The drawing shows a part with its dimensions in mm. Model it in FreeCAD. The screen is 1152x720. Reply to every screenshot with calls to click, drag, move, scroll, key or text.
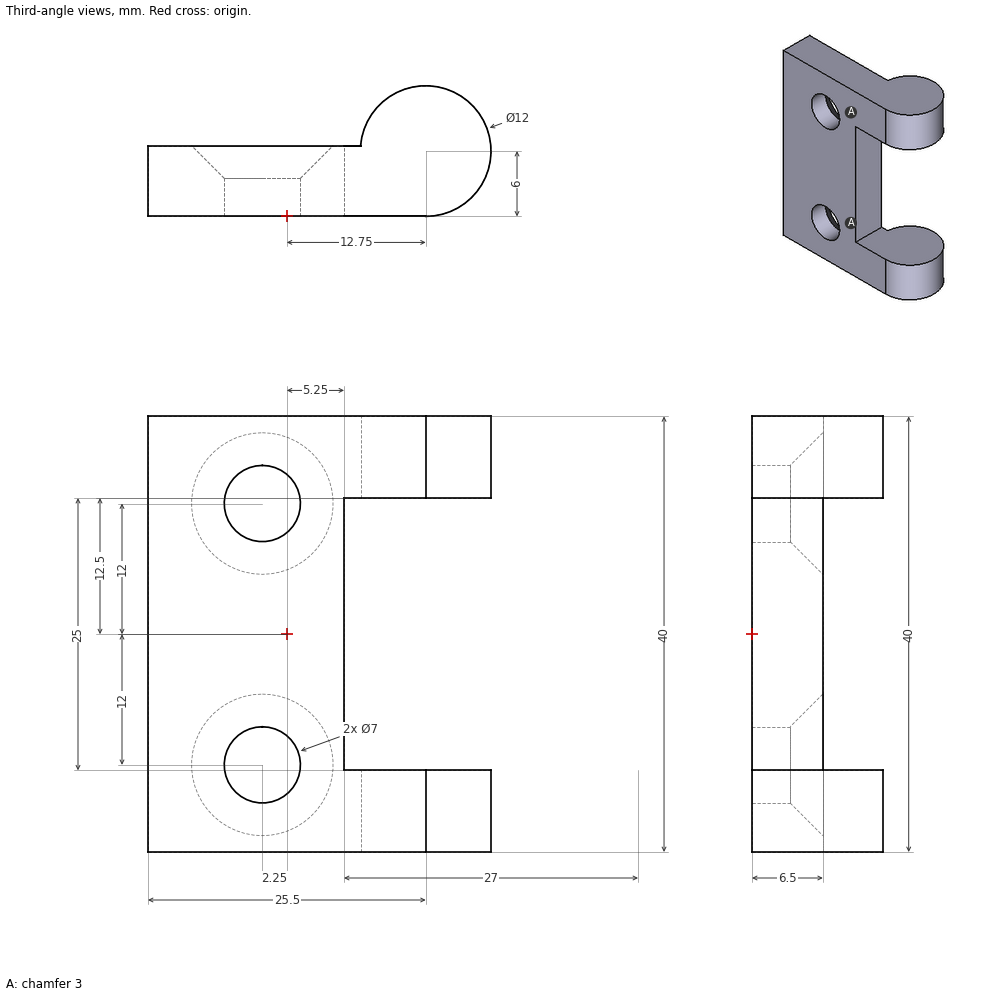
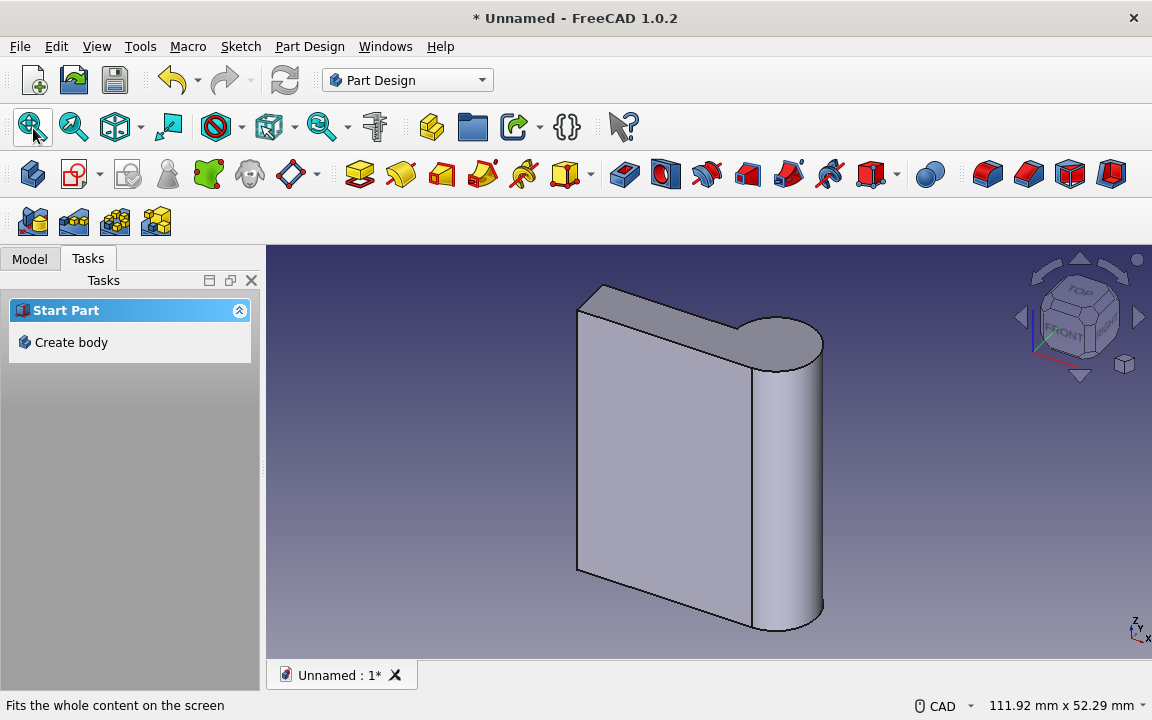
click(665, 431)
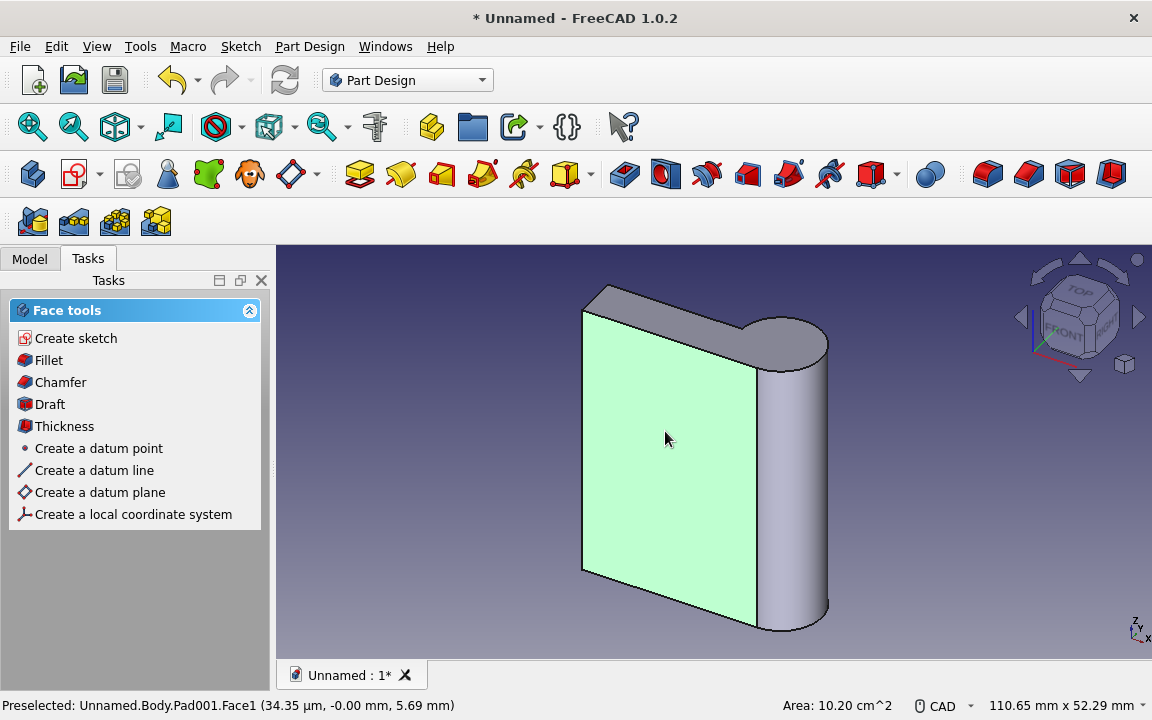
click(74, 174)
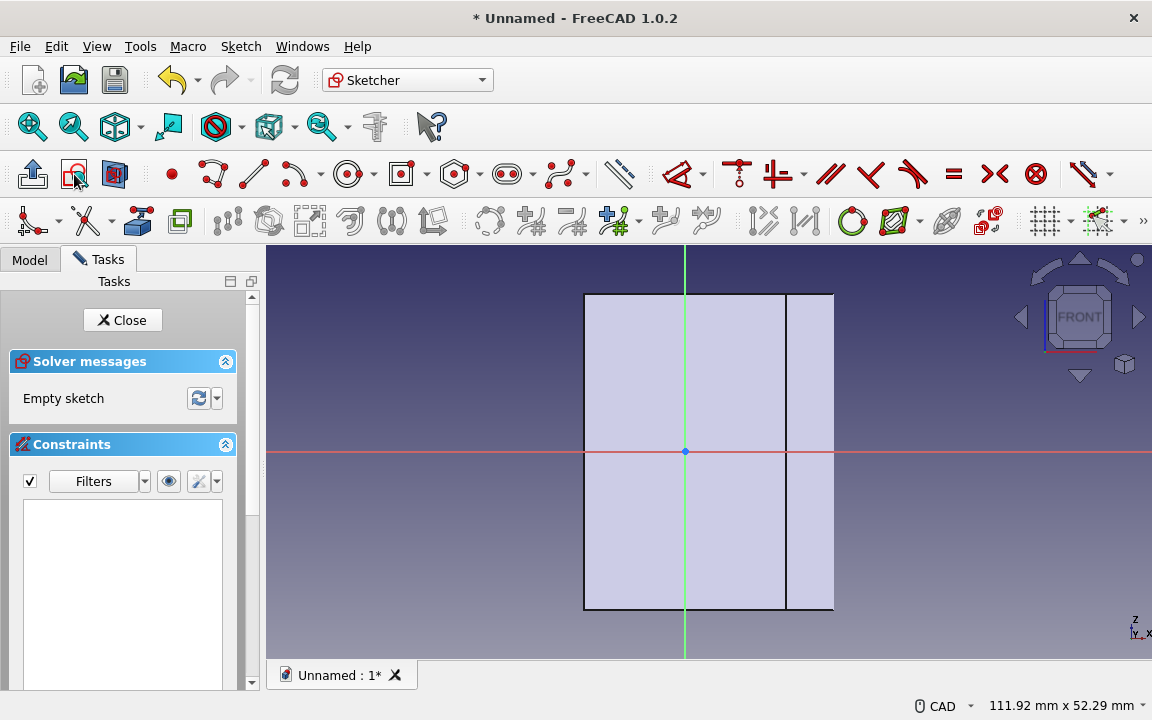
key(g)
key(r)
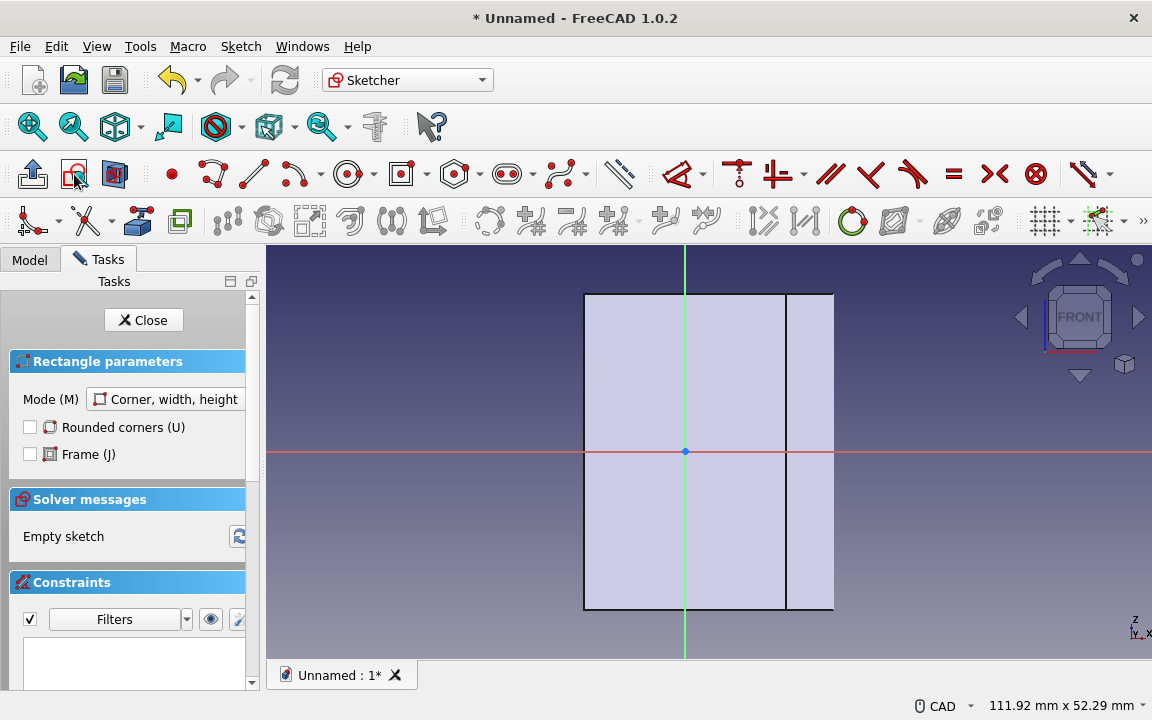
click(727, 353)
click(941, 551)
key(Escape)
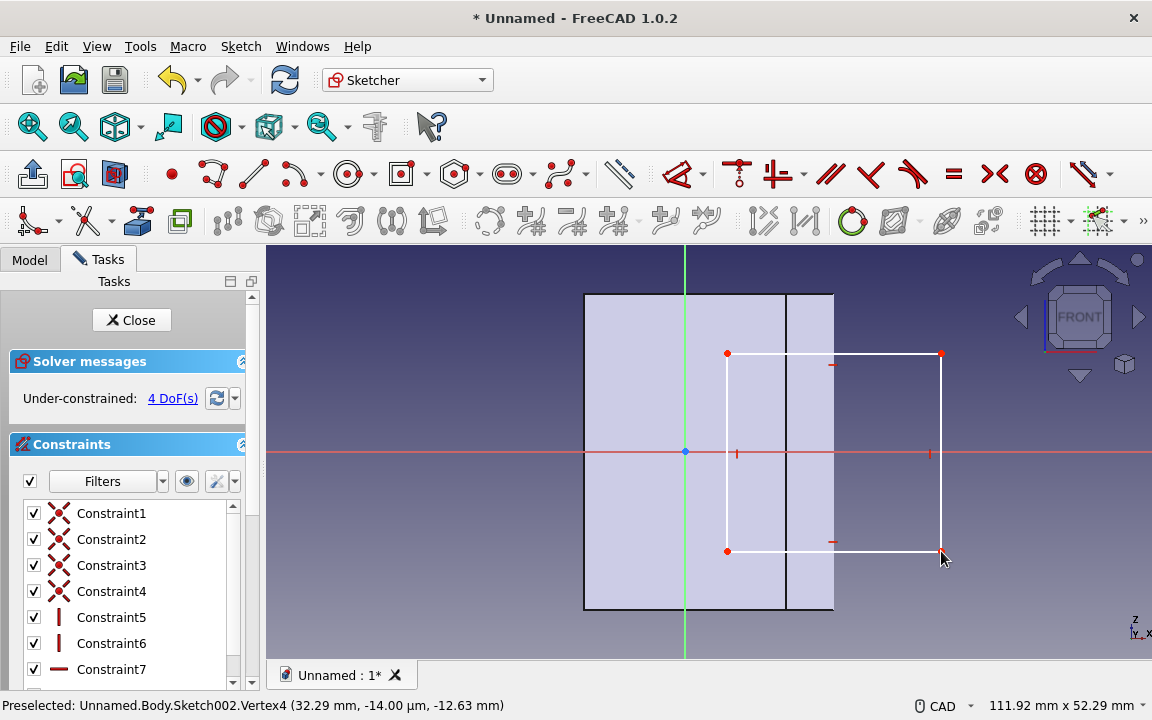
click(676, 174)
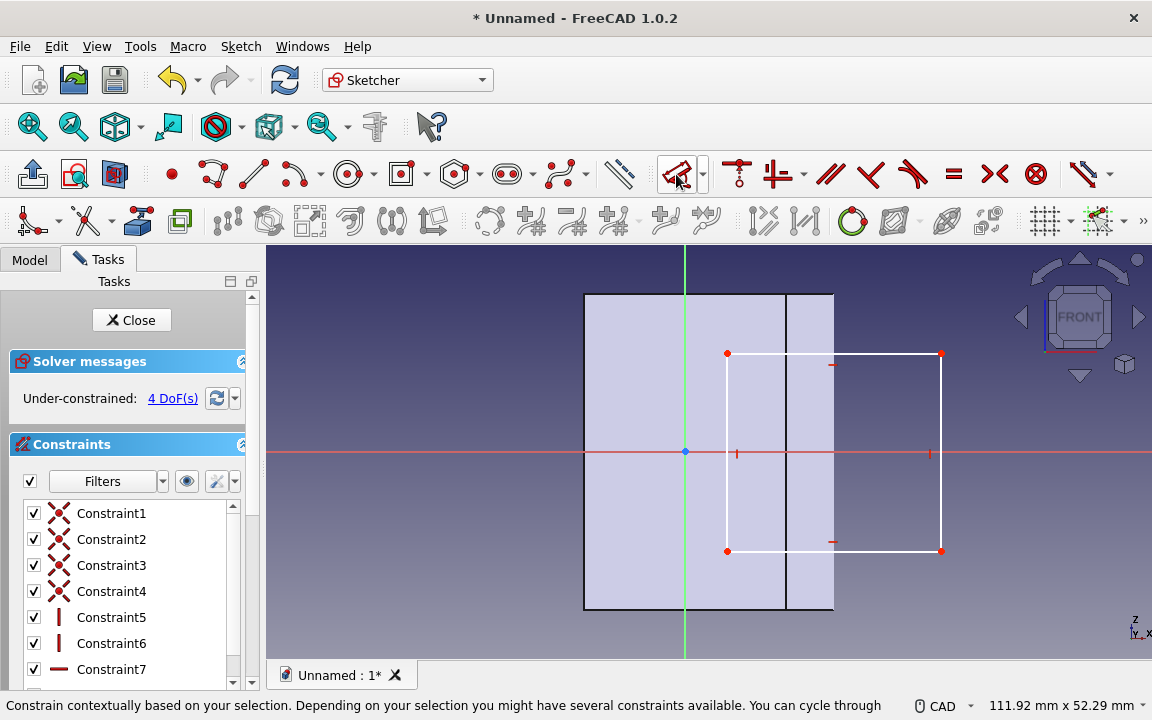
click(727, 413)
click(761, 407)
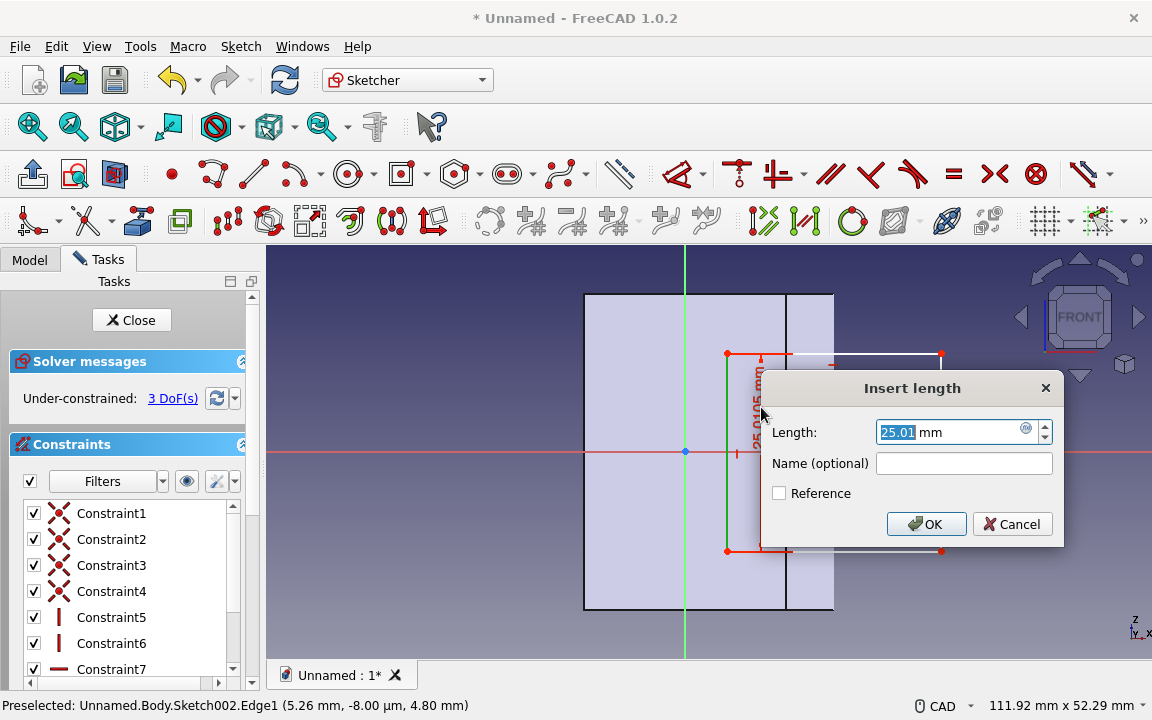
text(25)
key(Return)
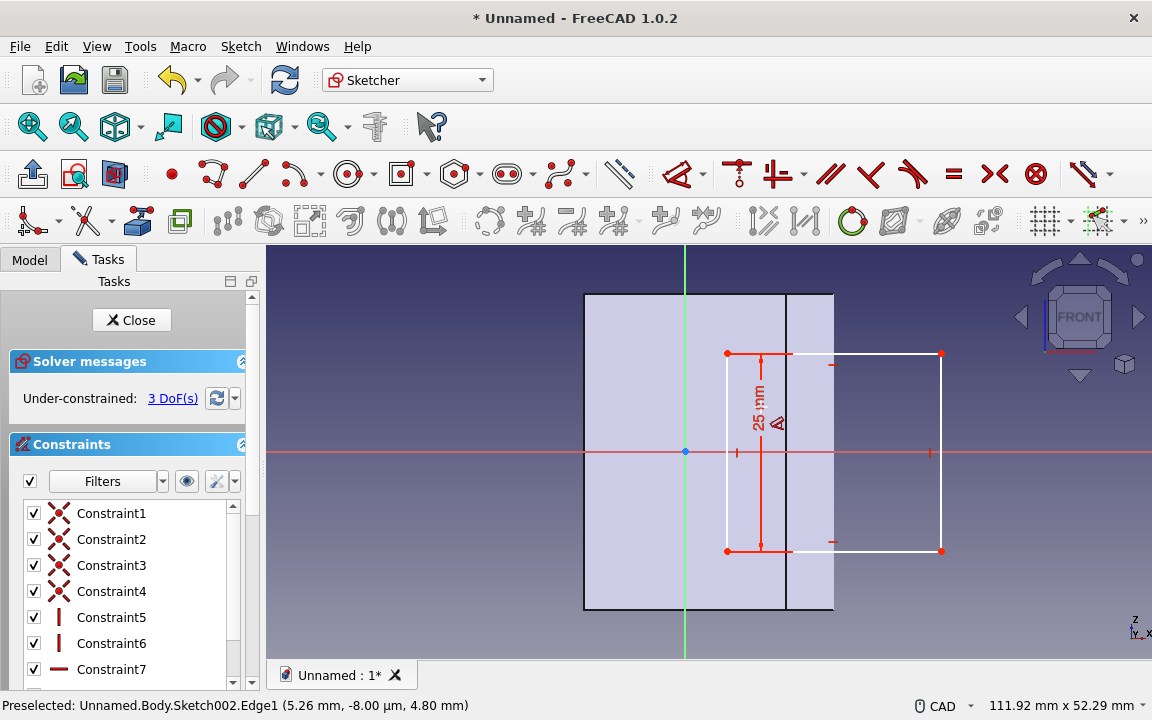
click(791, 552)
click(834, 586)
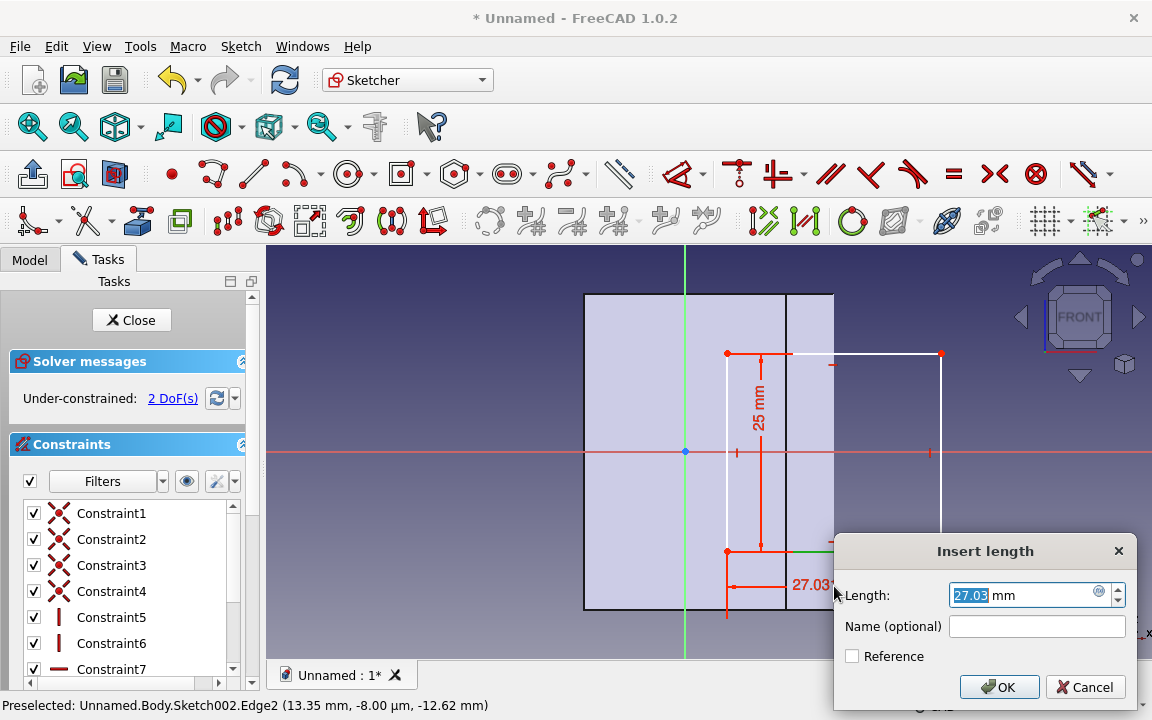
text(27)
key(Return)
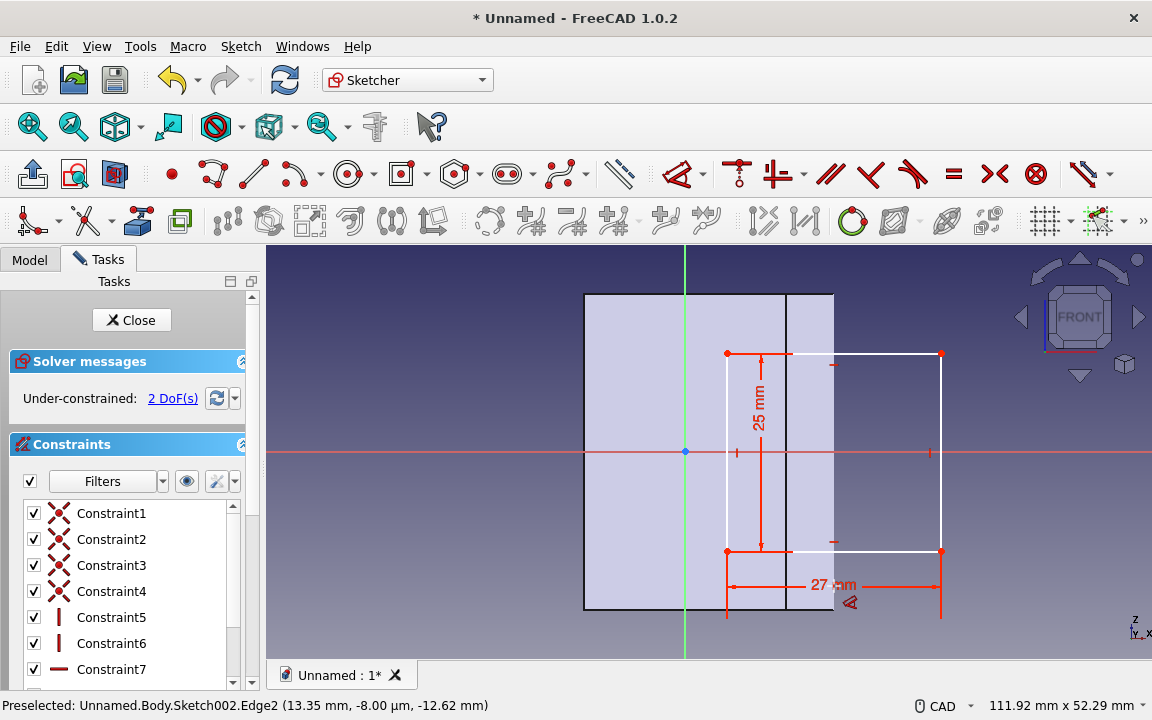
click(727, 354)
click(706, 320)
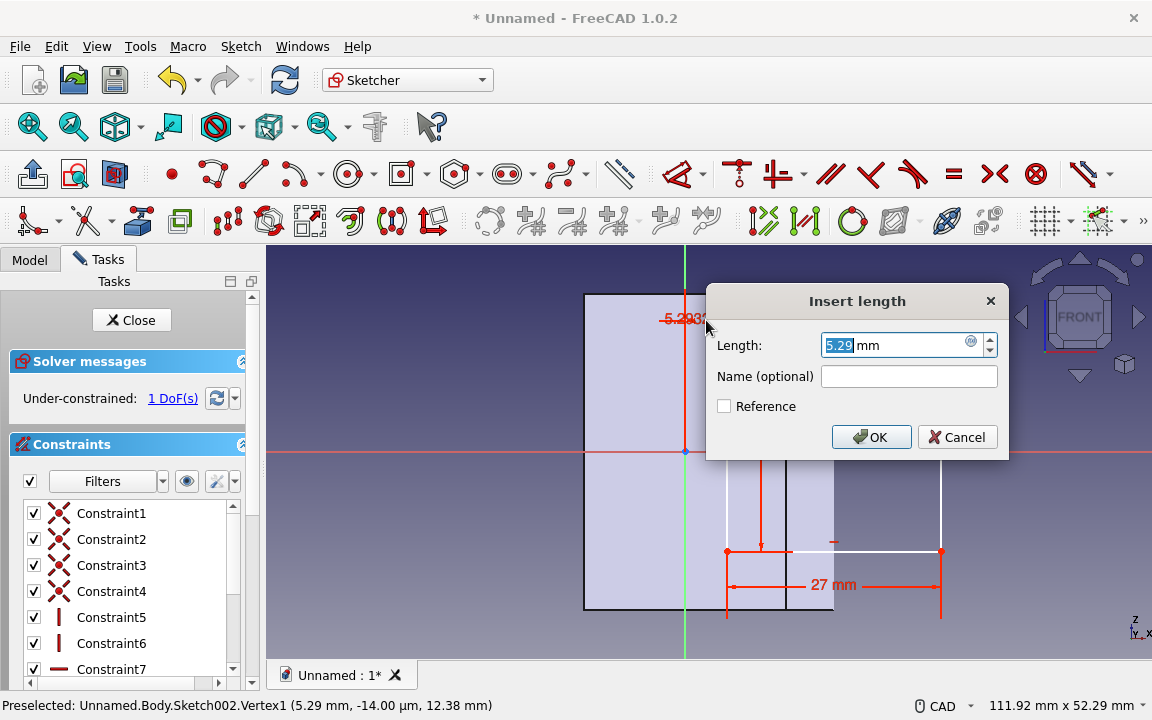
text(5.25)
key(Return)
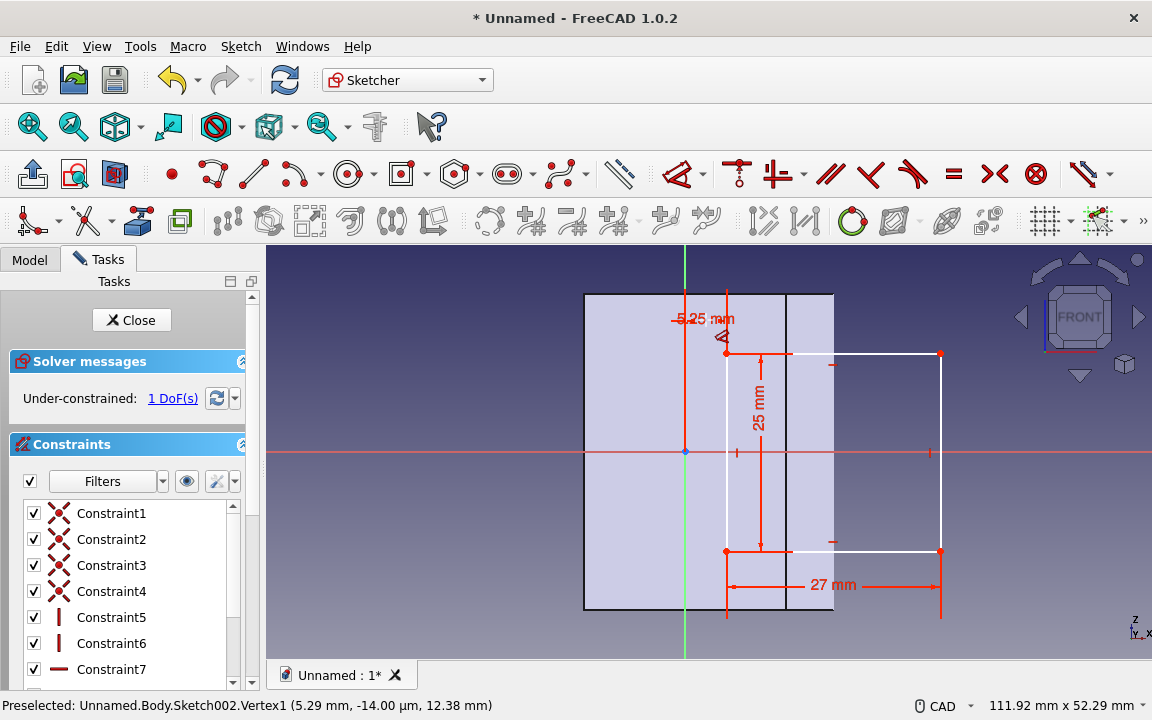
click(727, 354)
click(651, 403)